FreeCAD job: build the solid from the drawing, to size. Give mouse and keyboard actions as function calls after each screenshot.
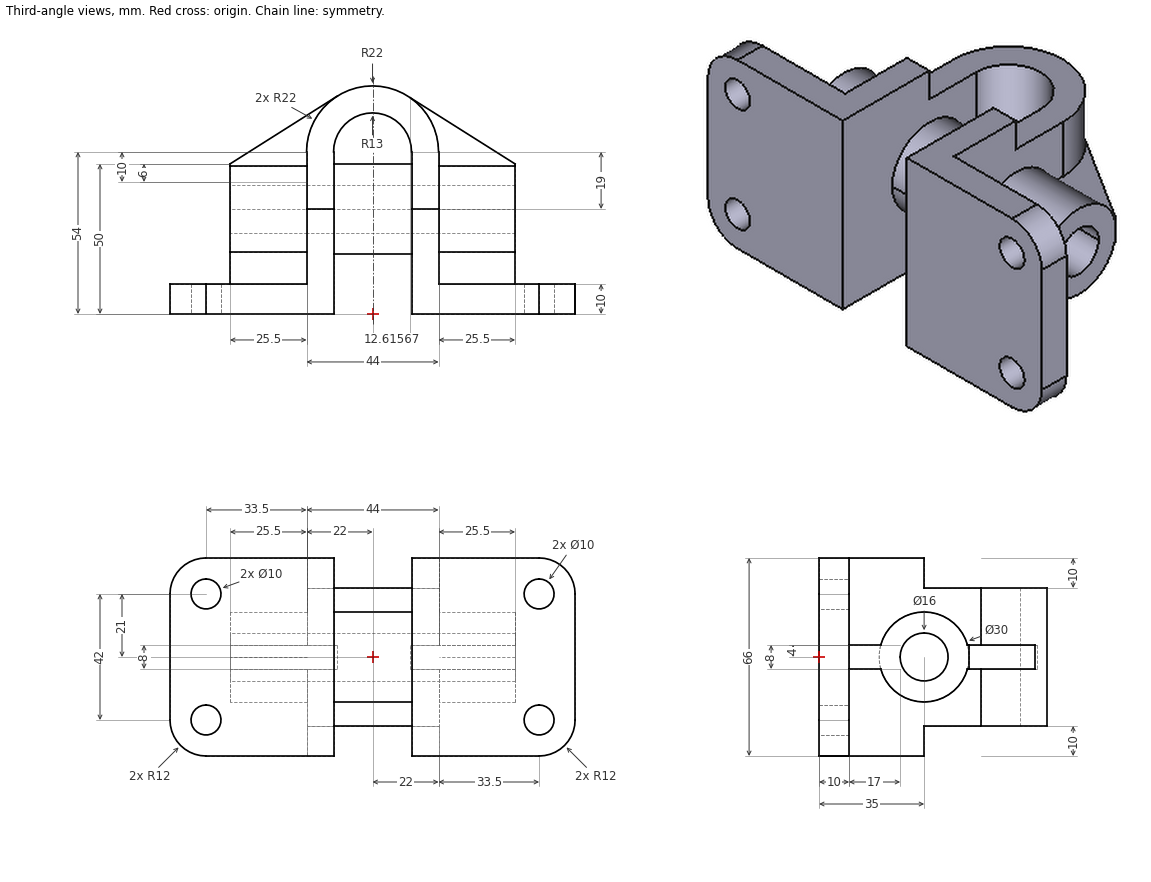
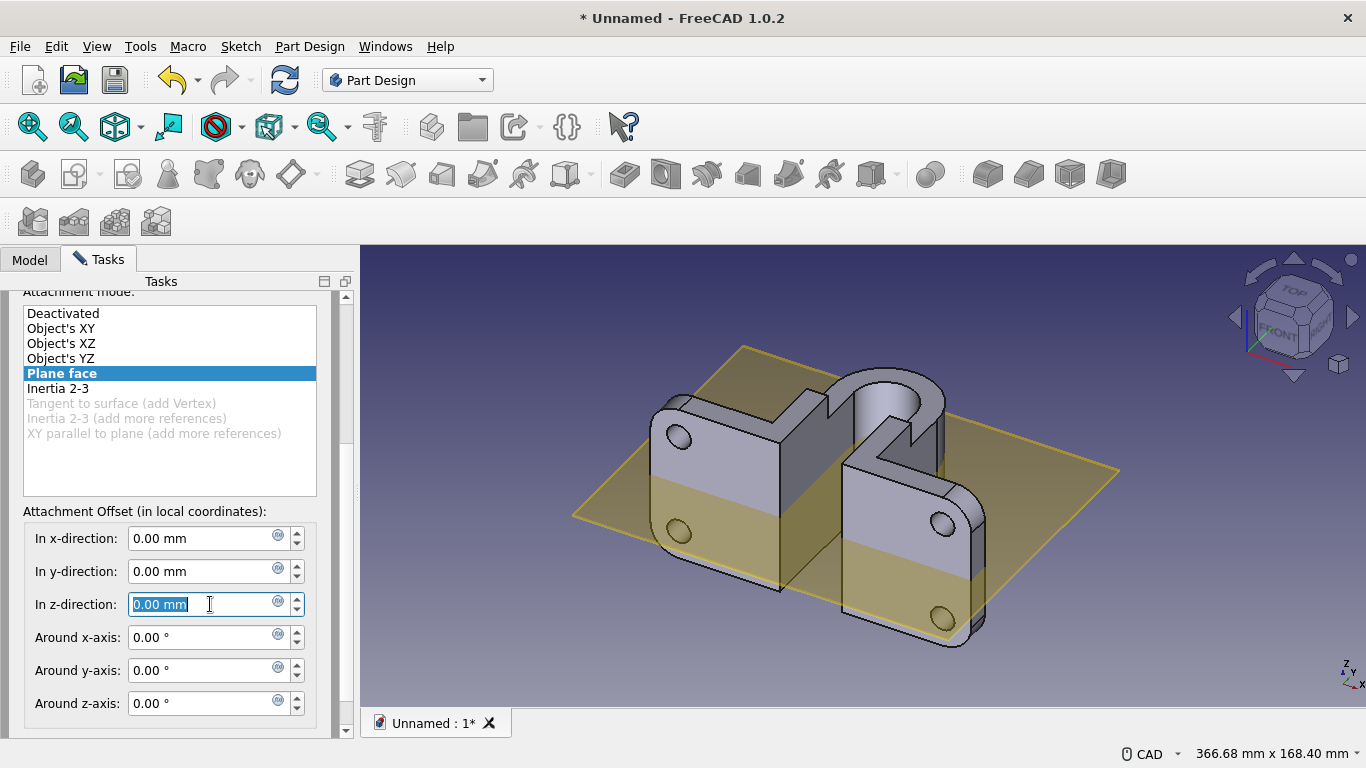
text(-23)
key(Tab)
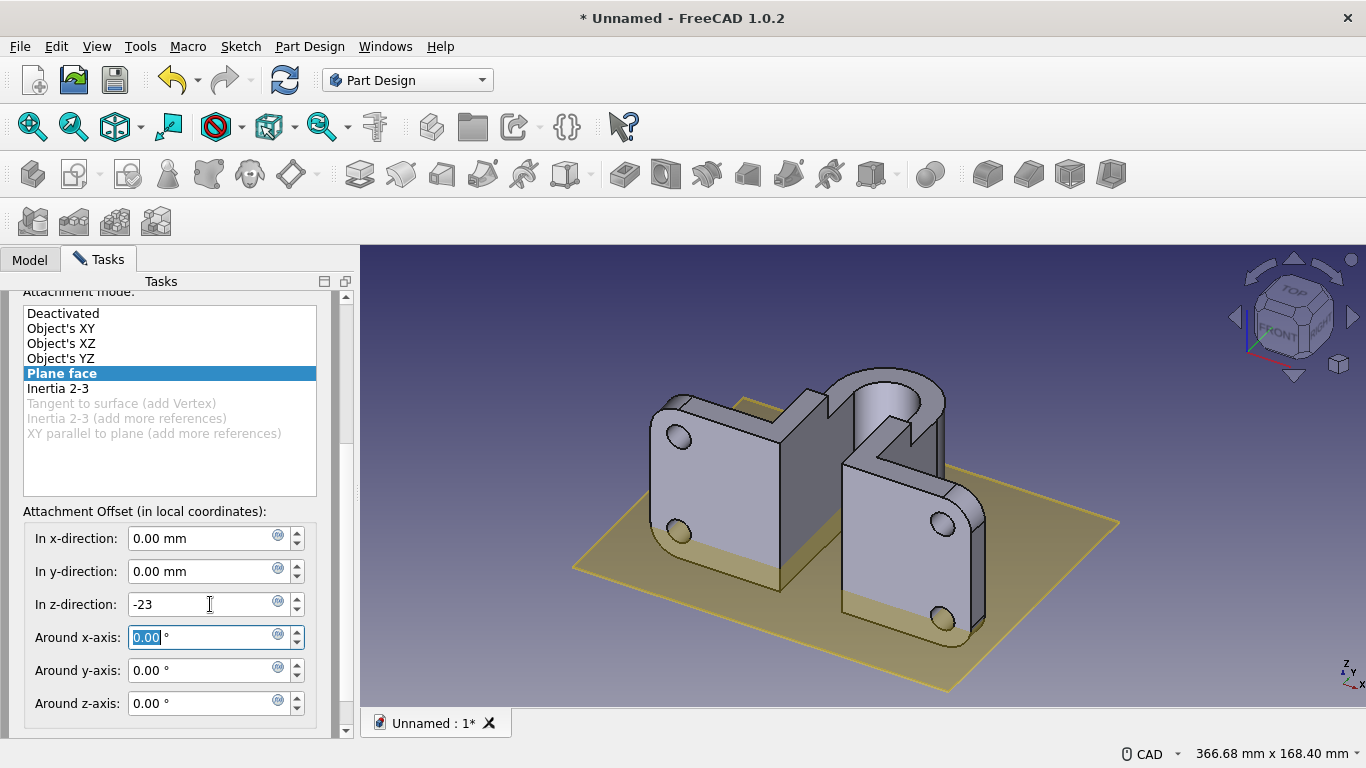
scroll(346, 514, up, 5)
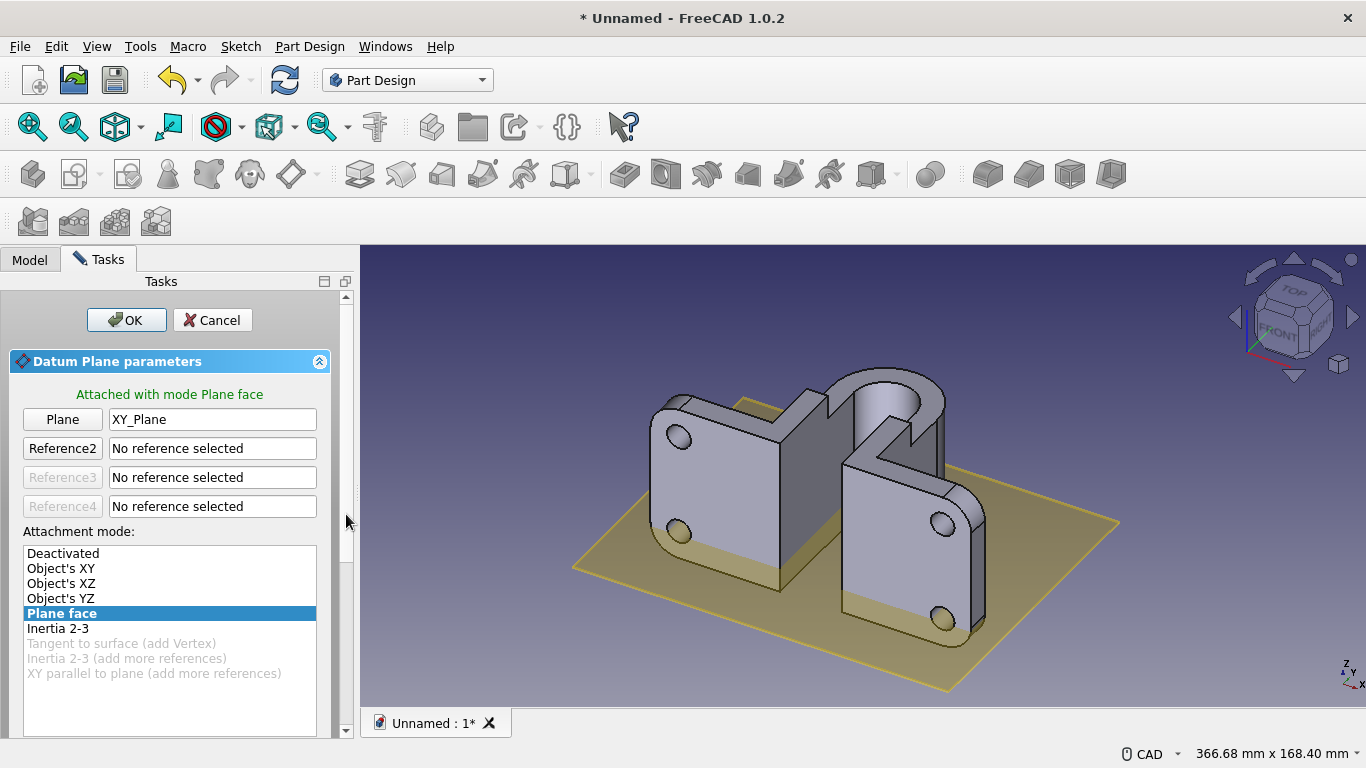
click(127, 320)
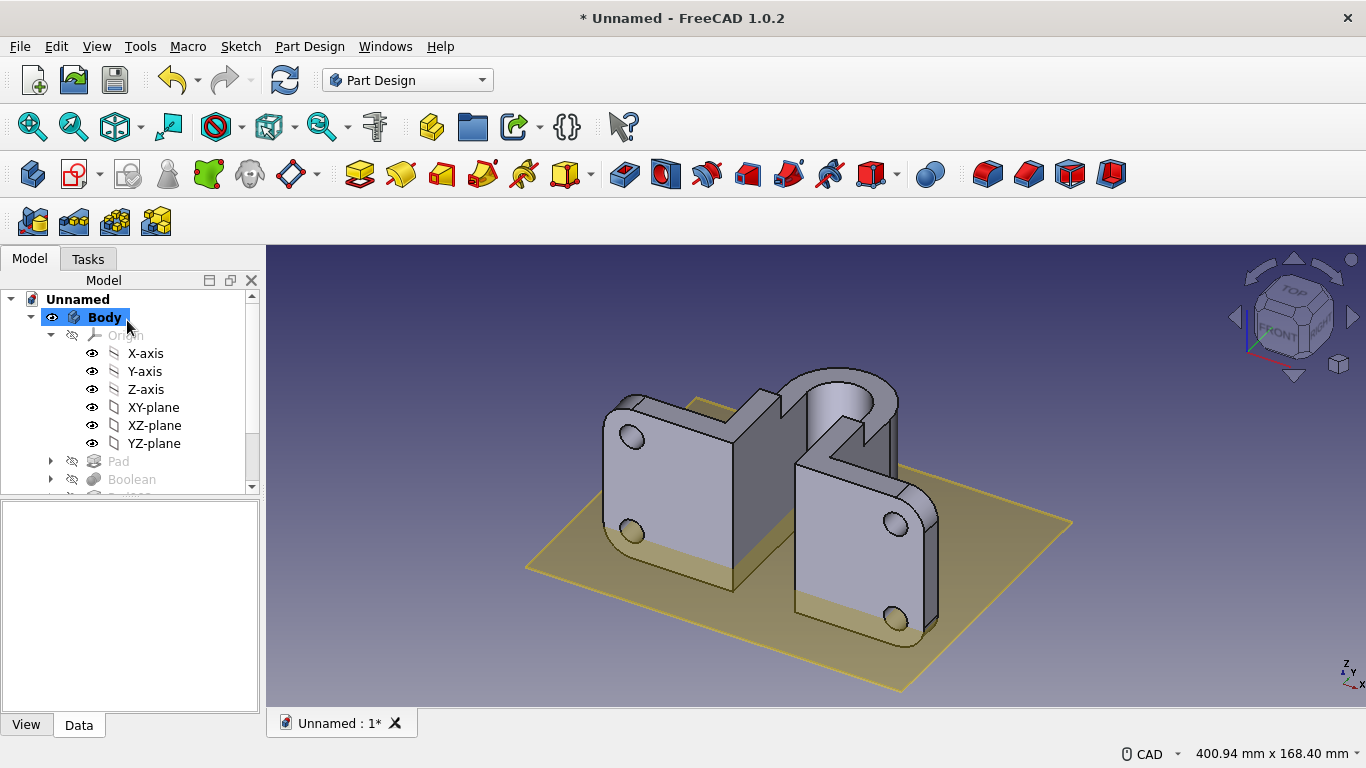
scroll(101, 385, down, 3)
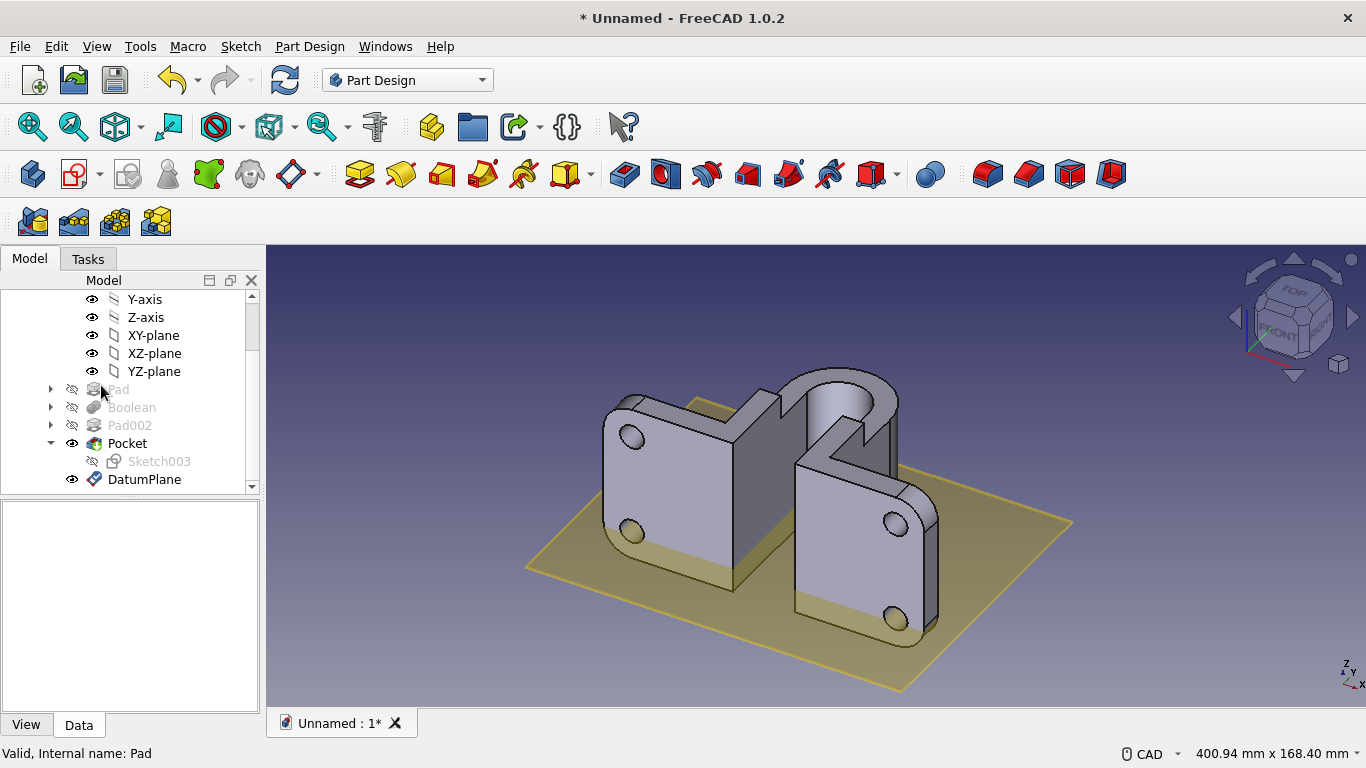
click(117, 479)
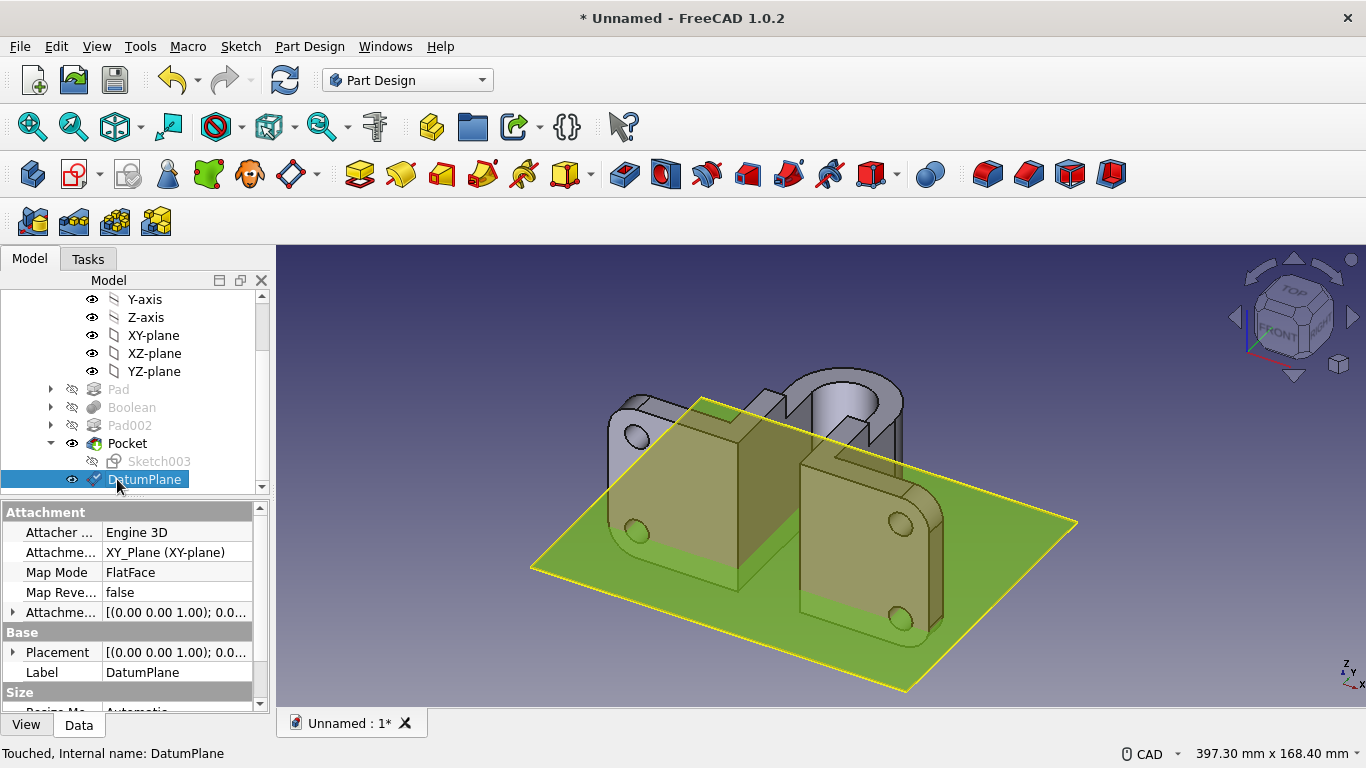
click(74, 174)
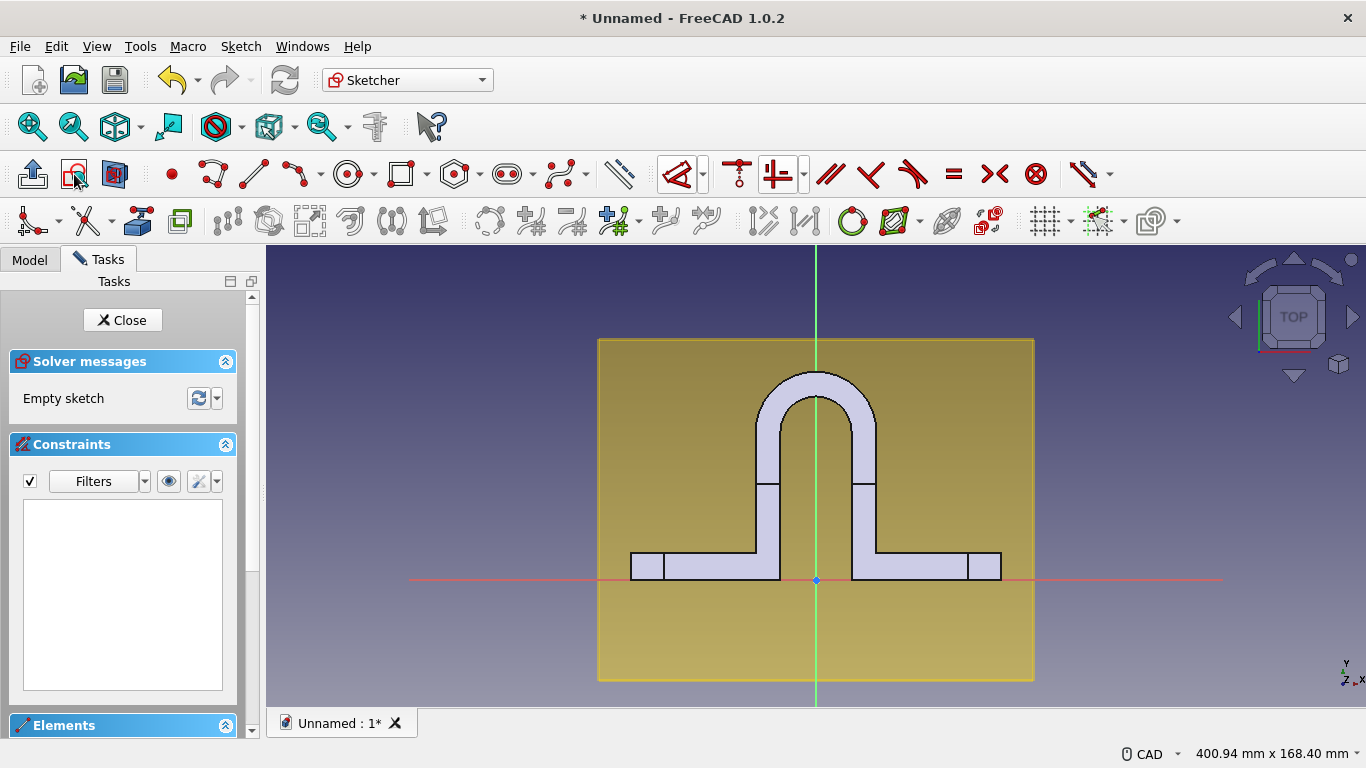
click(115, 174)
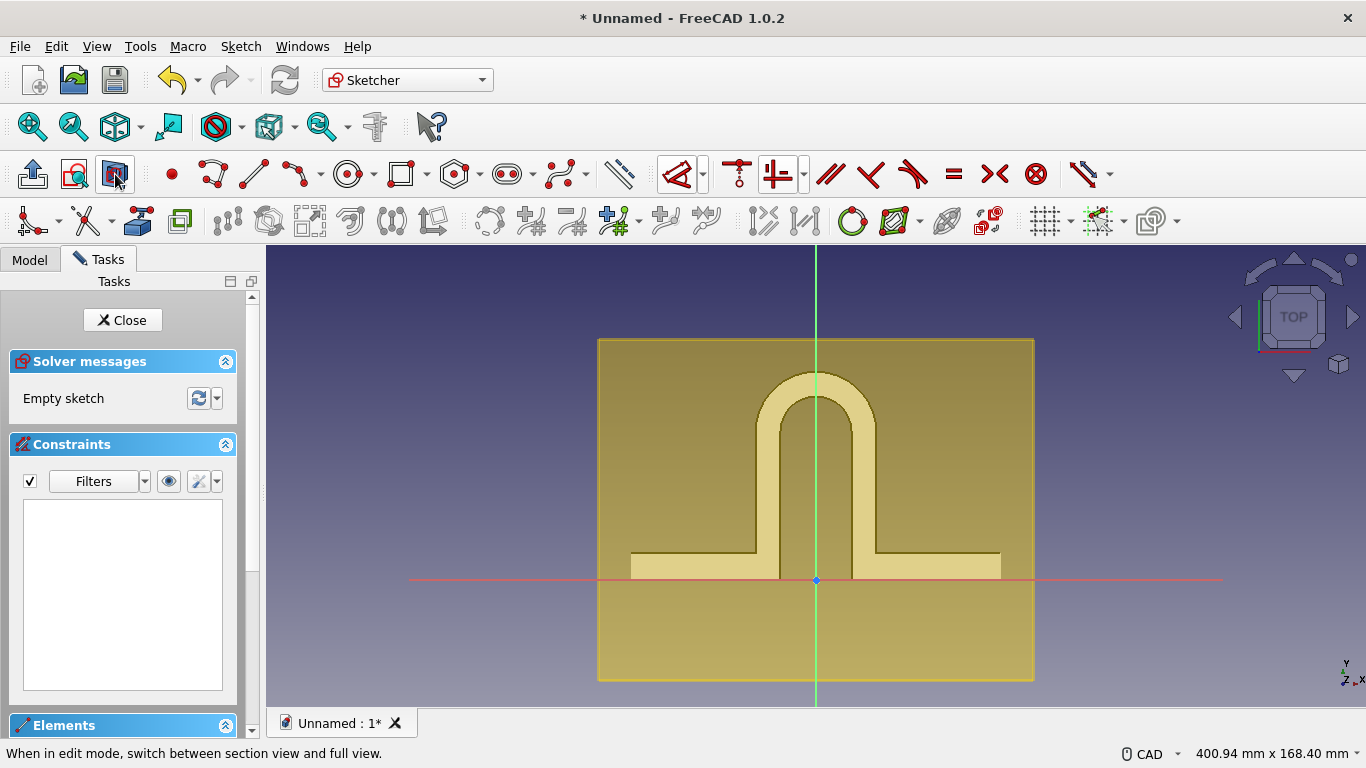
scroll(955, 476, up, 2)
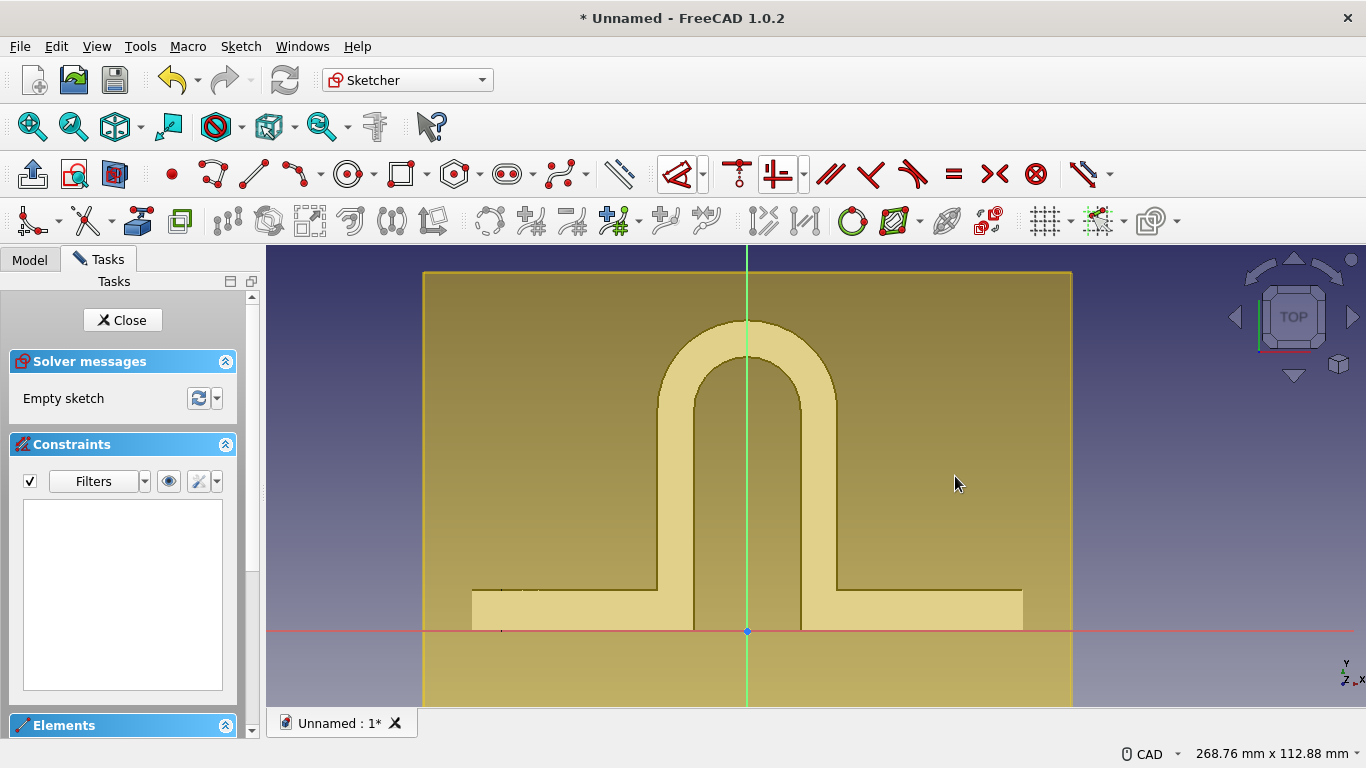
click(213, 174)